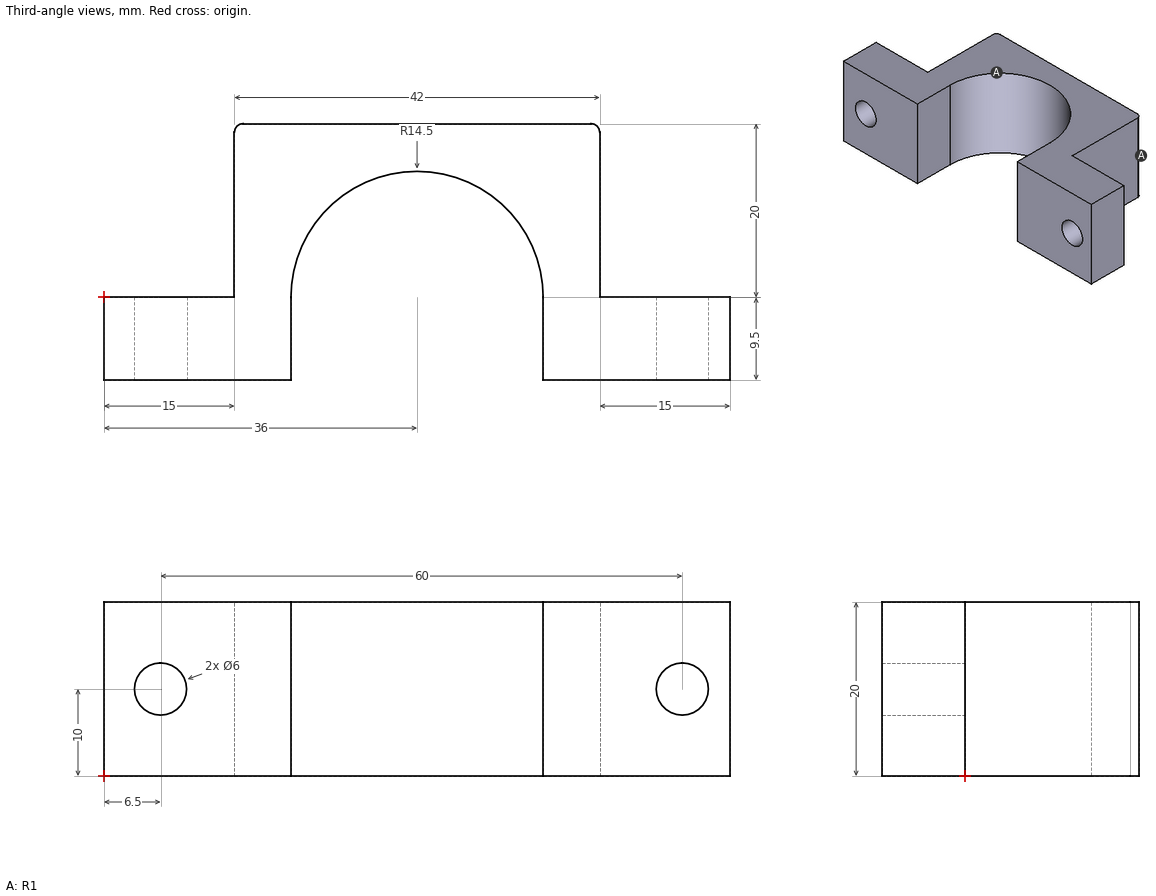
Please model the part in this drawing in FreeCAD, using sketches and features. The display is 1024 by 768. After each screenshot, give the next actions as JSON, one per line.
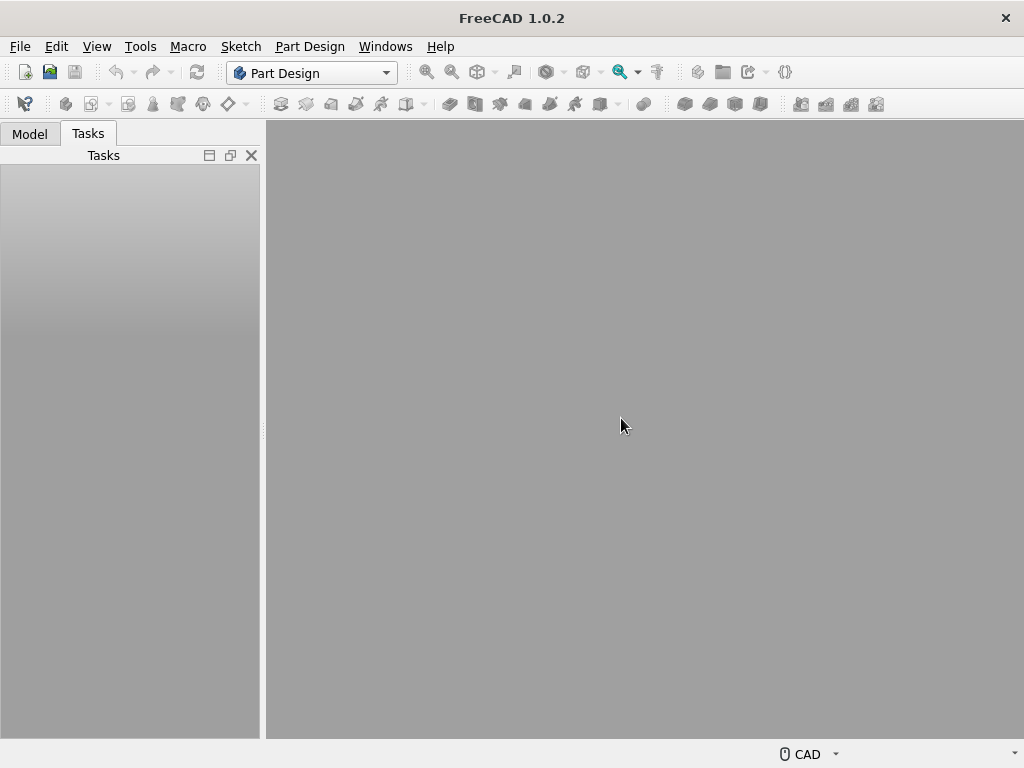
{"action": "left_click", "coordinate": [25, 72]}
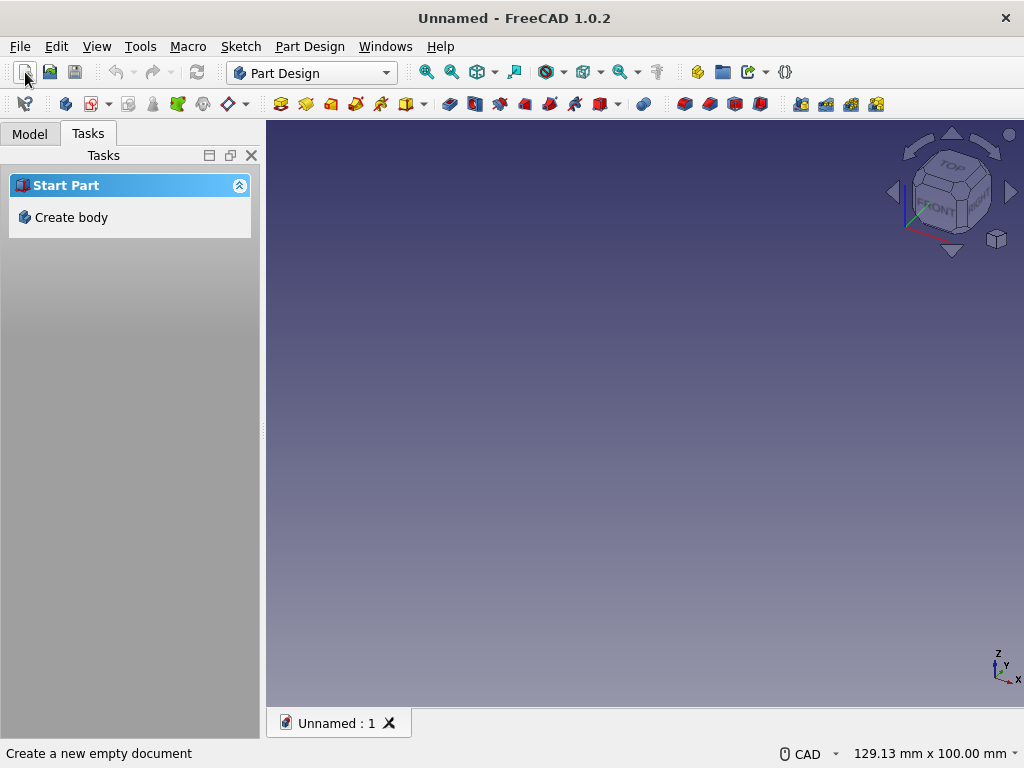
{"action": "left_click", "coordinate": [90, 104]}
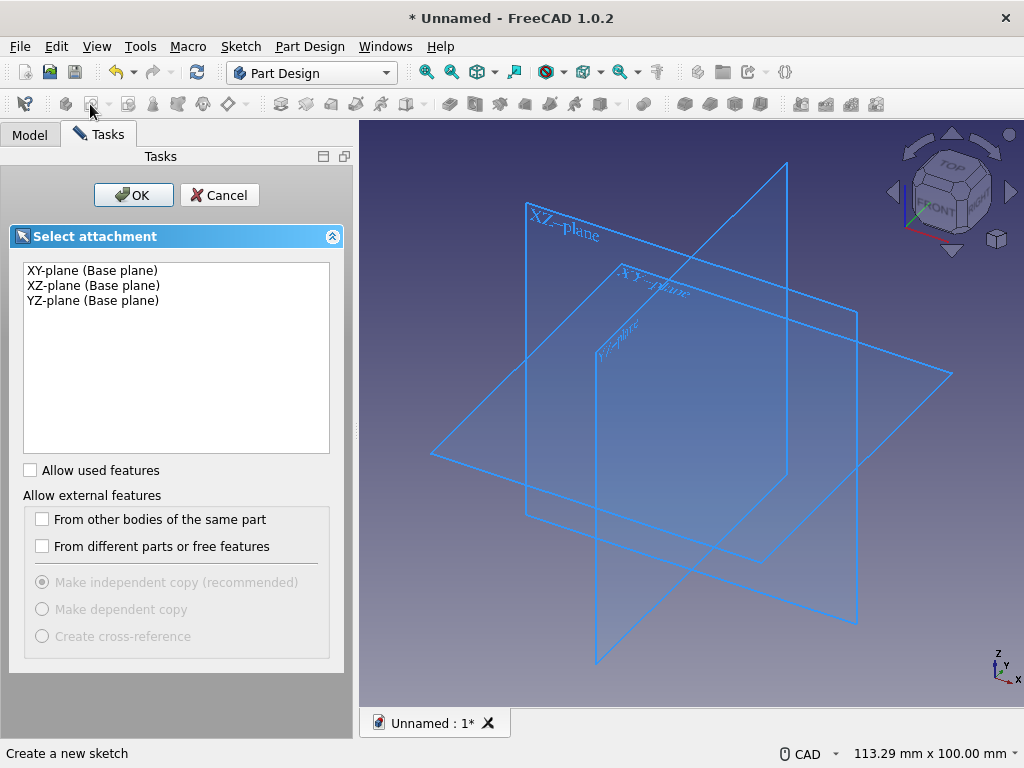
{"action": "left_click", "coordinate": [84, 270]}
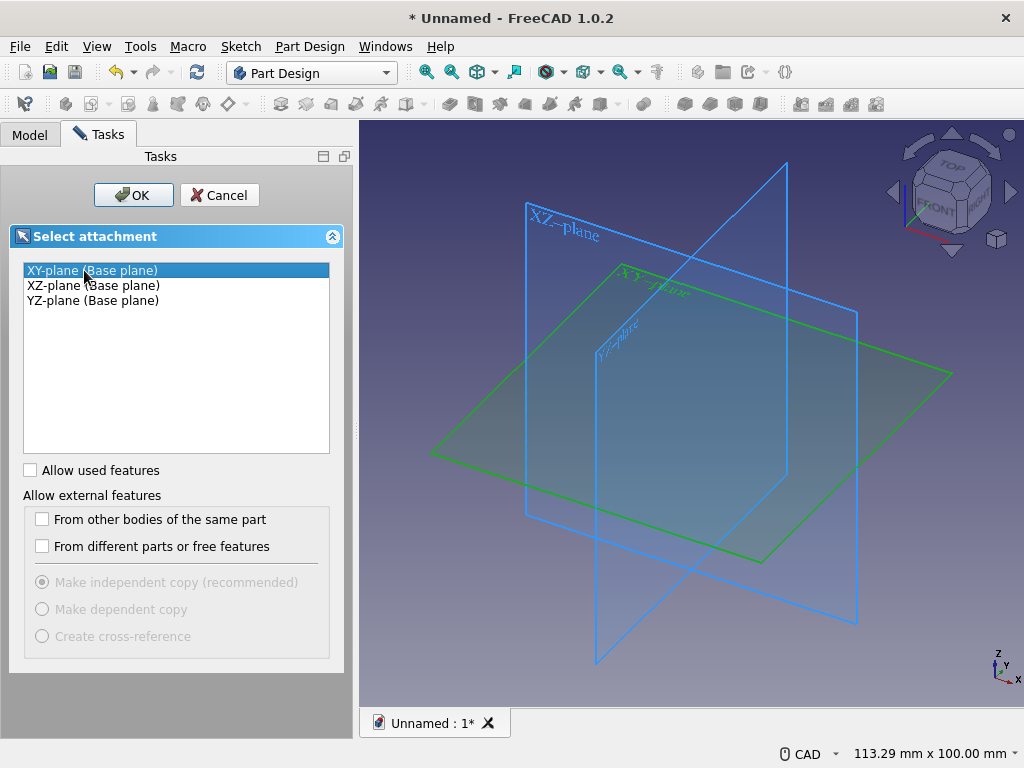
{"action": "left_click", "coordinate": [134, 195]}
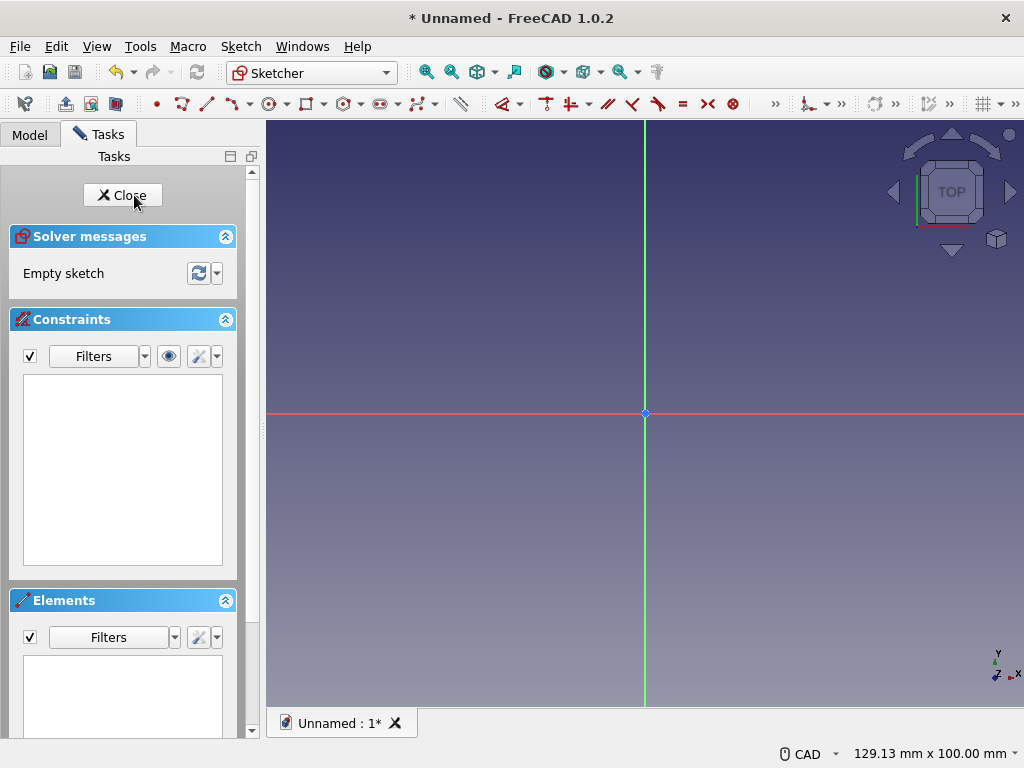
{"action": "scroll", "coordinate": [294, 476], "scroll_direction": "down", "scroll_amount": 2}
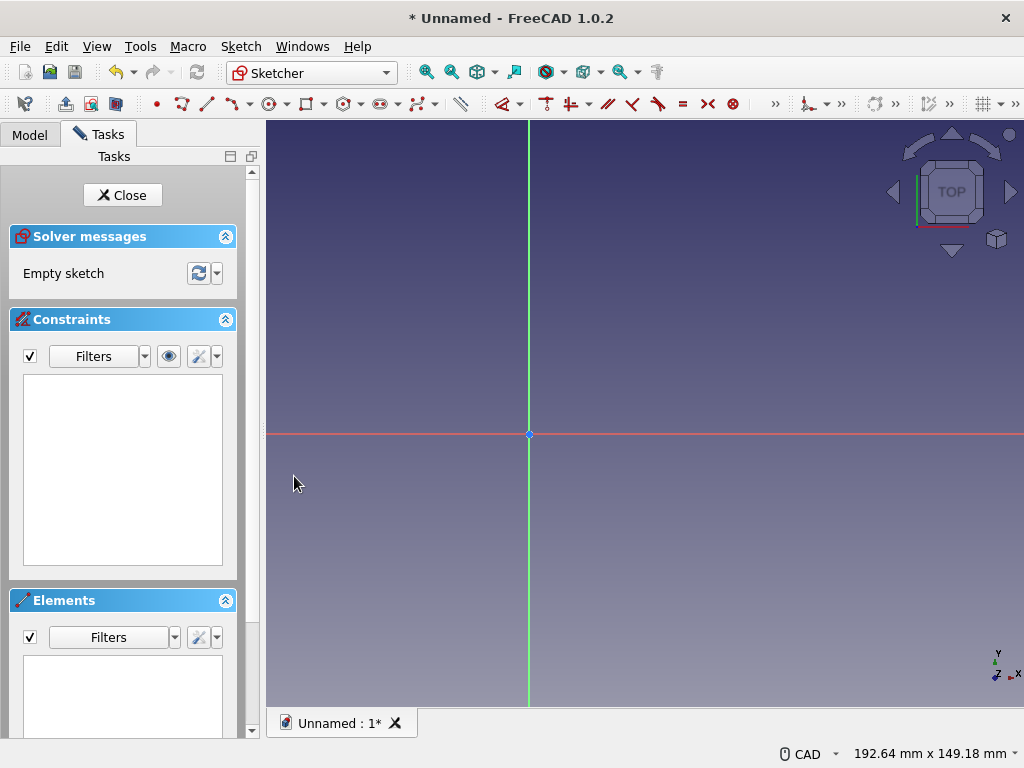
{"action": "scroll", "coordinate": [859, 414], "scroll_direction": "up", "scroll_amount": 2}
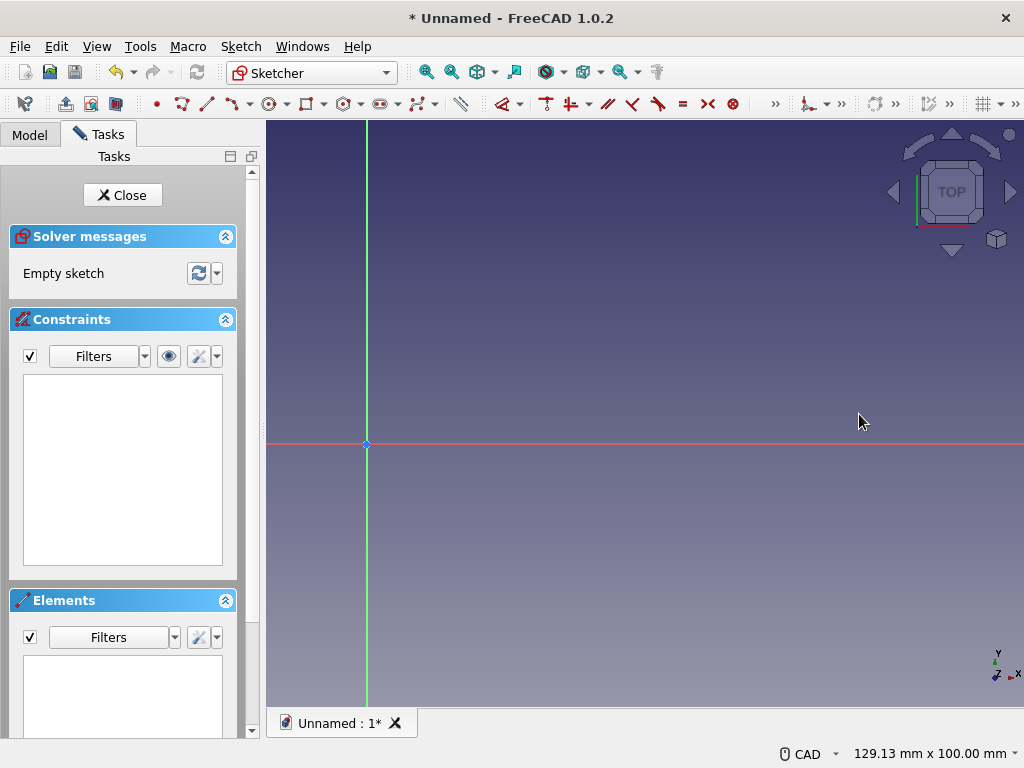
{"action": "left_click", "coordinate": [182, 104]}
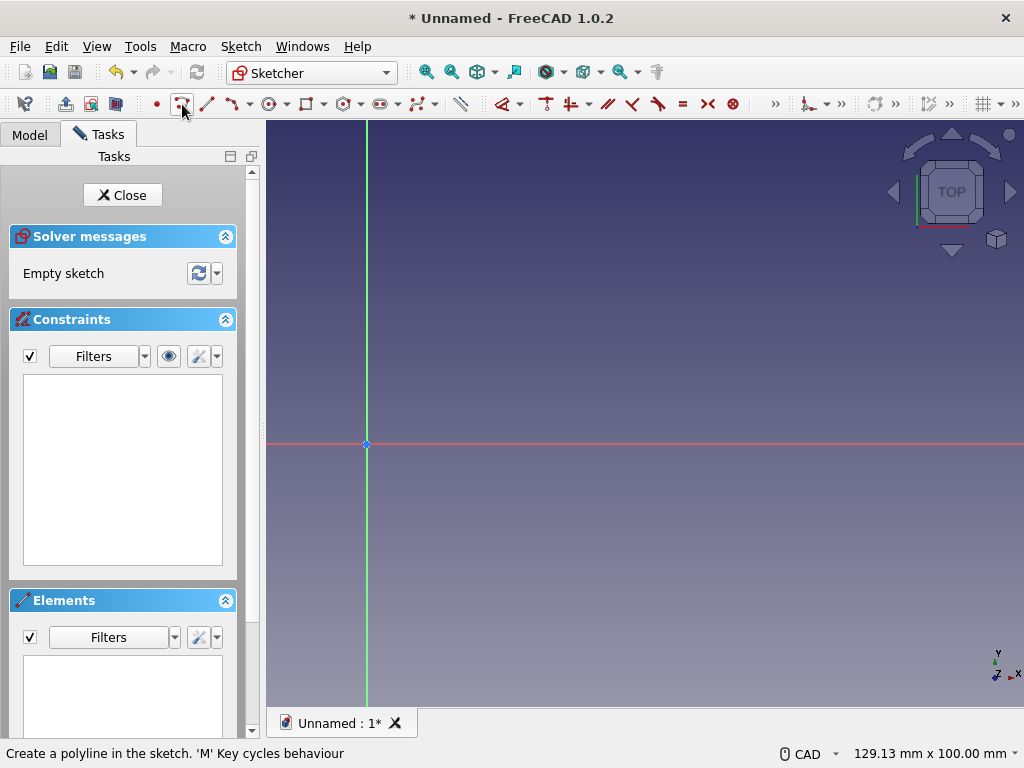
{"action": "left_click", "coordinate": [663, 444]}
{"action": "left_click", "coordinate": [663, 500]}
{"action": "left_click", "coordinate": [789, 500]}
{"action": "left_click", "coordinate": [789, 444]}
{"action": "left_click", "coordinate": [701, 435]}
{"action": "left_click", "coordinate": [701, 327]}
{"action": "left_click", "coordinate": [455, 327]}
{"action": "left_click", "coordinate": [455, 444]}
{"action": "left_click", "coordinate": [367, 444]}
{"action": "left_click", "coordinate": [376, 500]}
{"action": "left_click", "coordinate": [493, 500]}
{"action": "left_click", "coordinate": [493, 444]}
{"action": "right_click", "coordinate": [493, 444]}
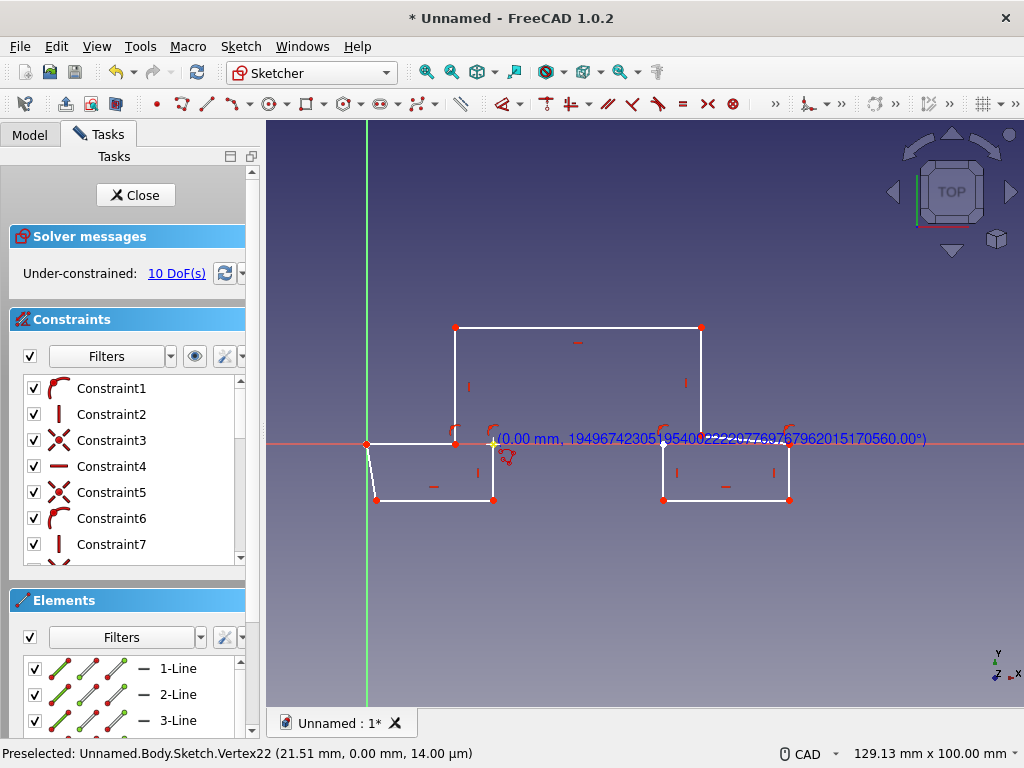
{"action": "key", "text": "g 3 a"}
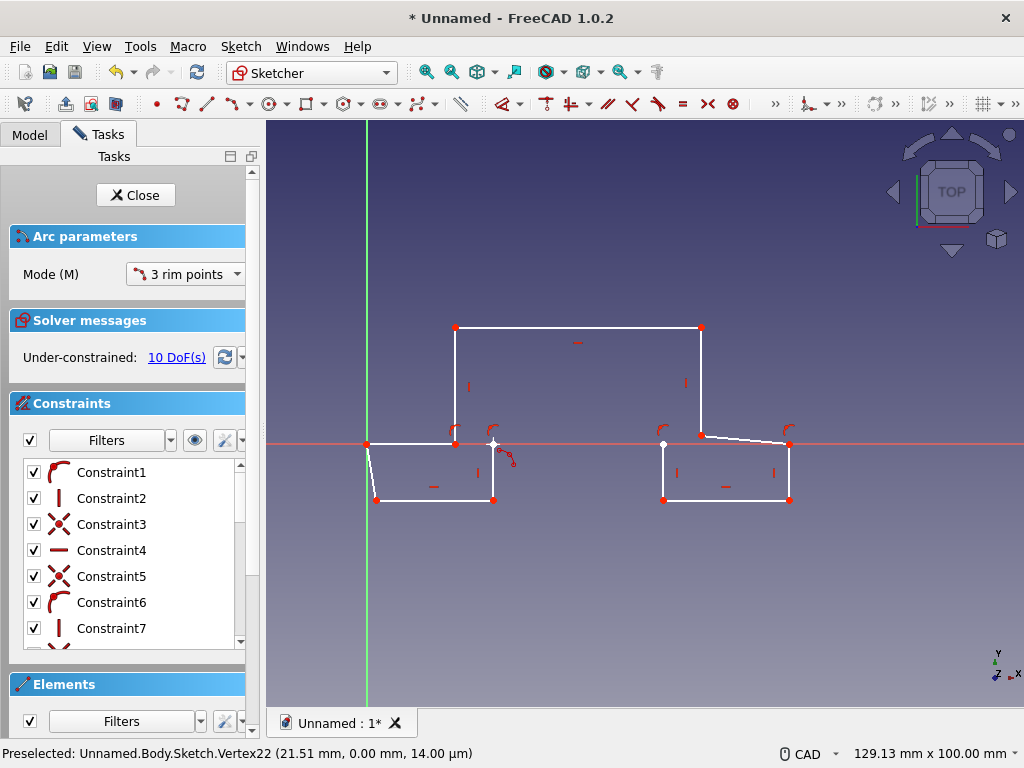
{"action": "left_click", "coordinate": [493, 444]}
{"action": "left_click", "coordinate": [663, 444]}
{"action": "left_click", "coordinate": [578, 359]}
{"action": "key", "text": "Escape"}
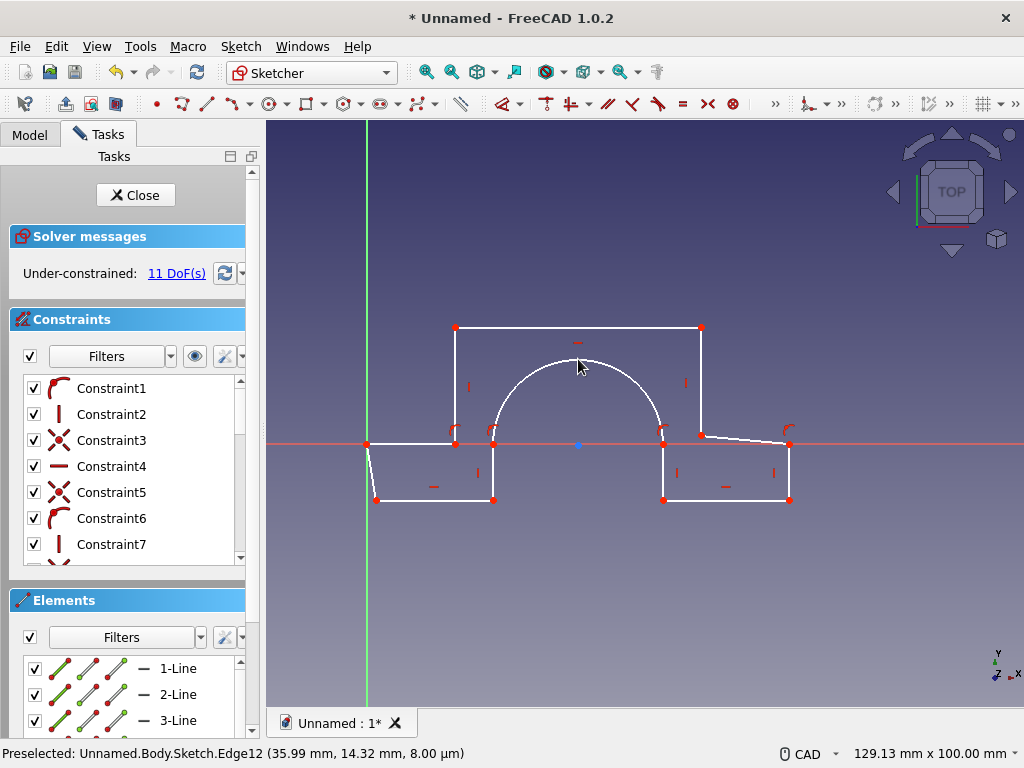
{"action": "left_click", "coordinate": [663, 461]}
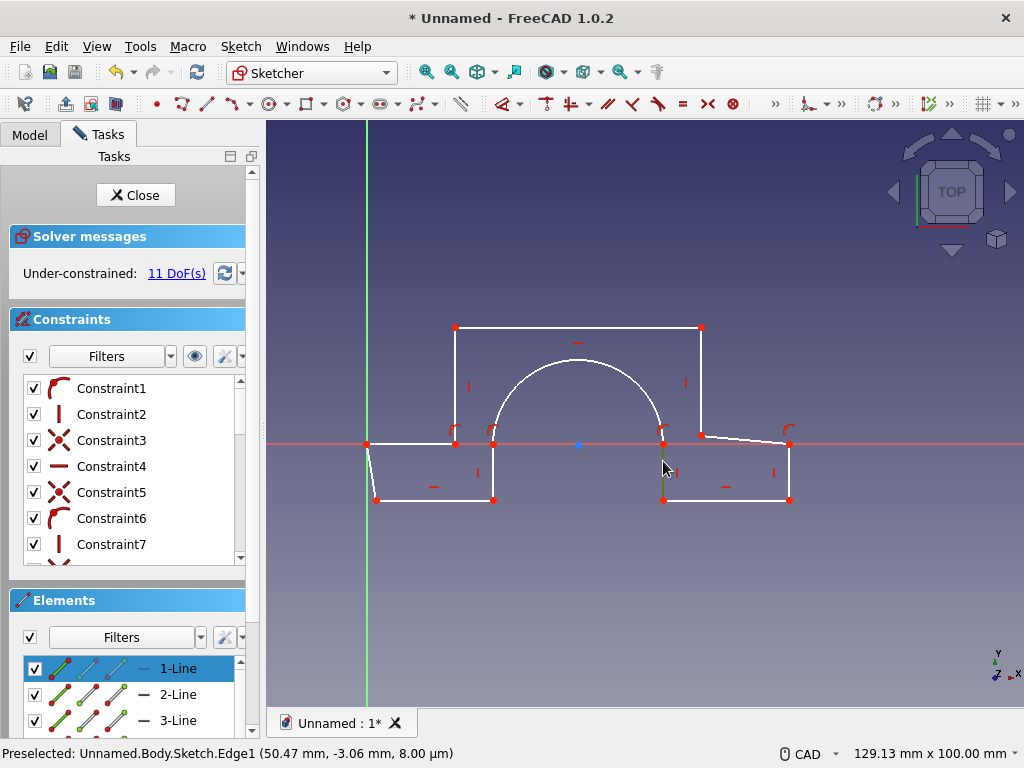
{"action": "left_click", "coordinate": [628, 376]}